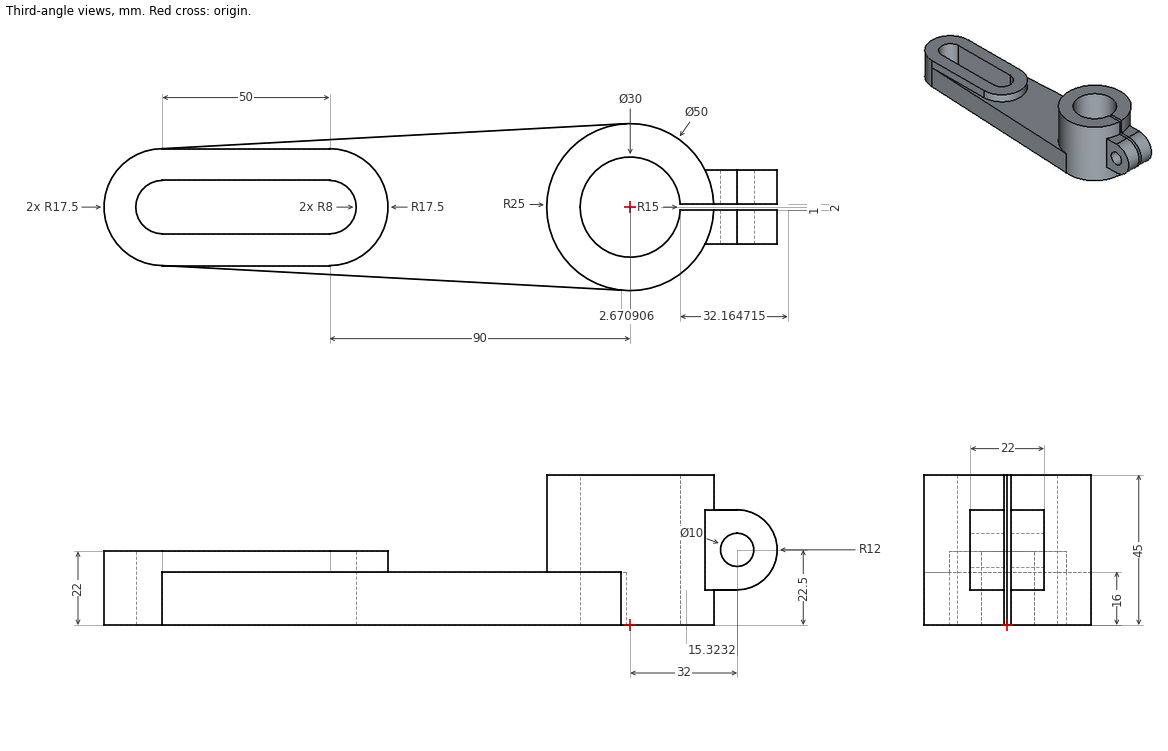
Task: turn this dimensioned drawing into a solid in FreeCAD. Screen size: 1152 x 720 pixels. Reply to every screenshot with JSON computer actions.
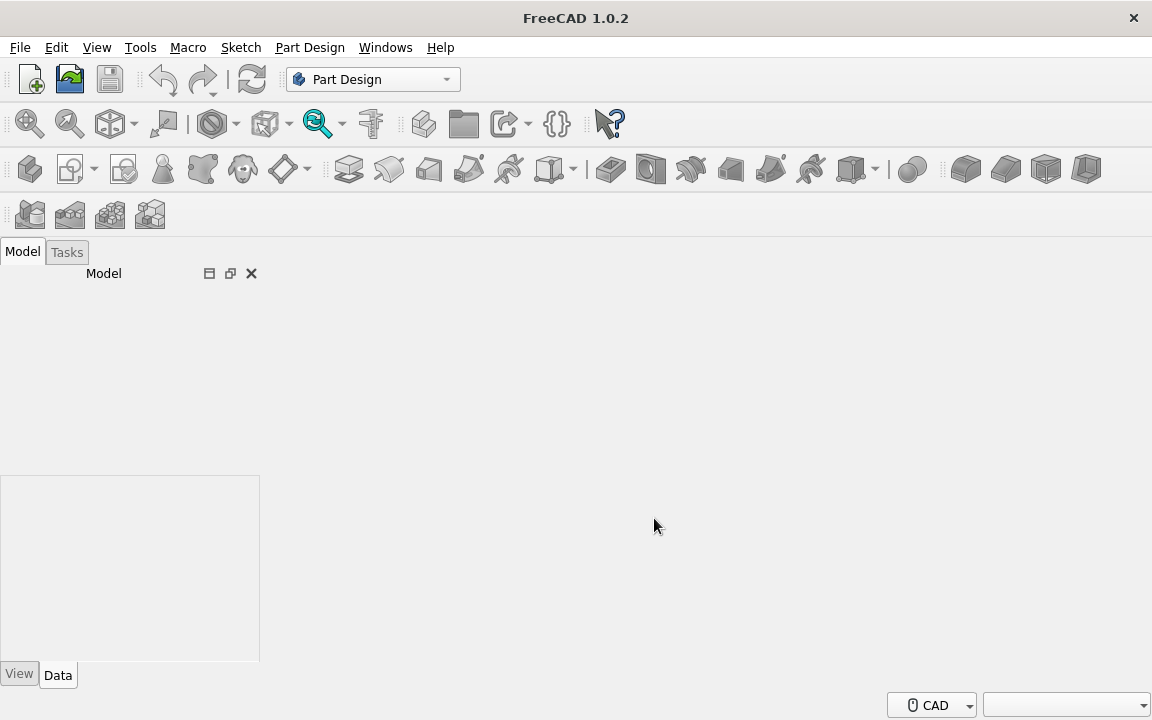
{"action": "left_click", "coordinate": [30, 80]}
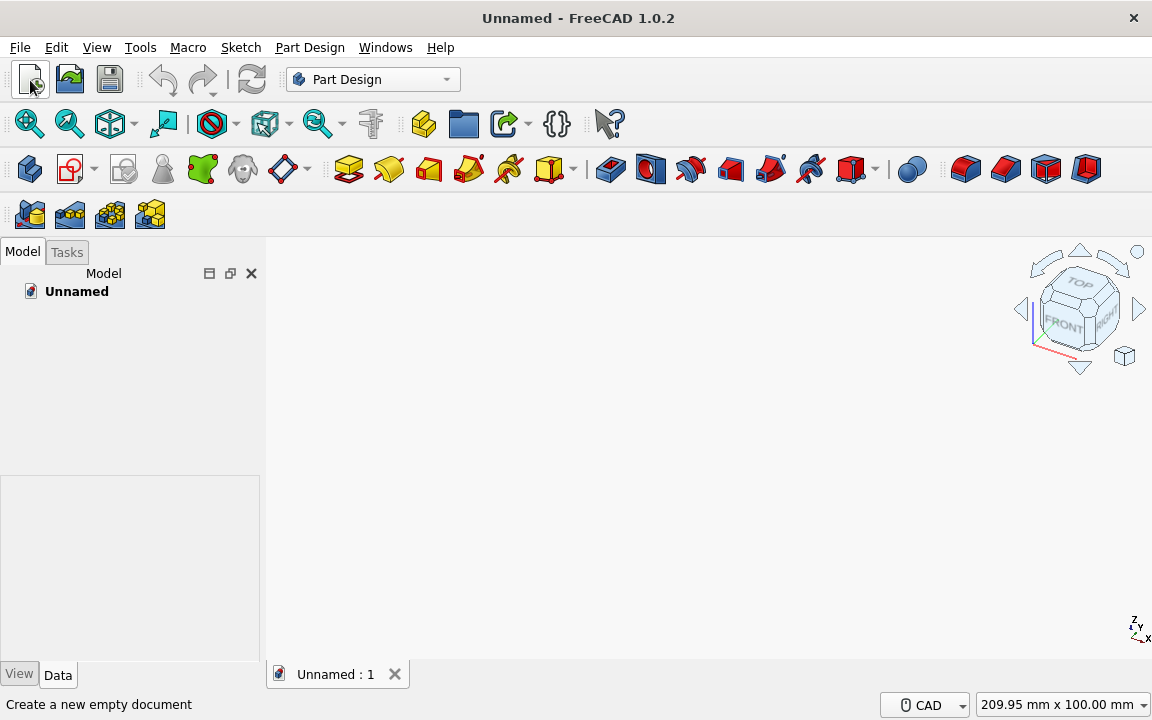
{"action": "left_click", "coordinate": [70, 170]}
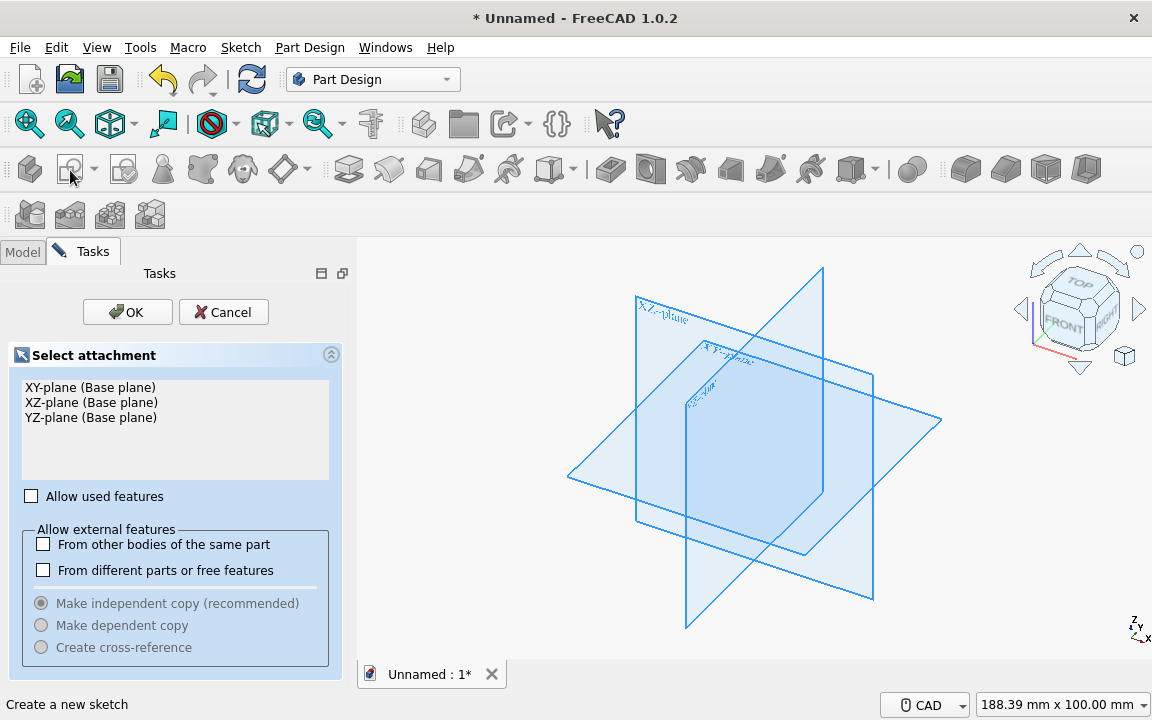
{"action": "left_click", "coordinate": [82, 388]}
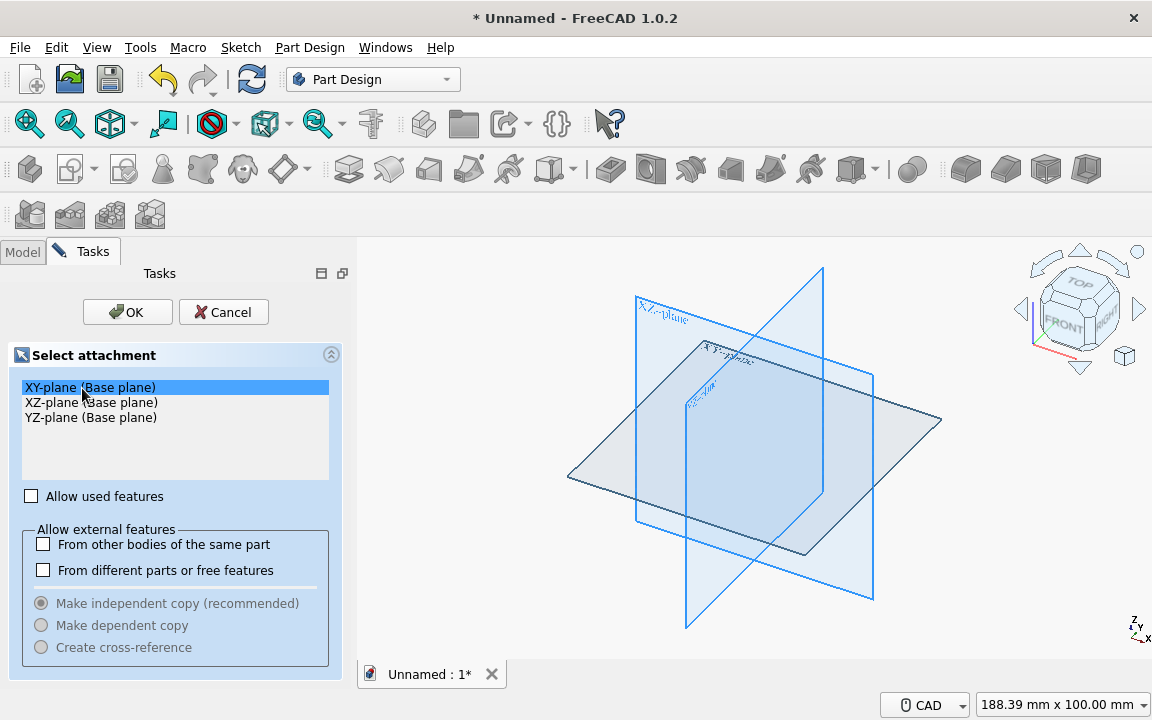
{"action": "left_click", "coordinate": [128, 312]}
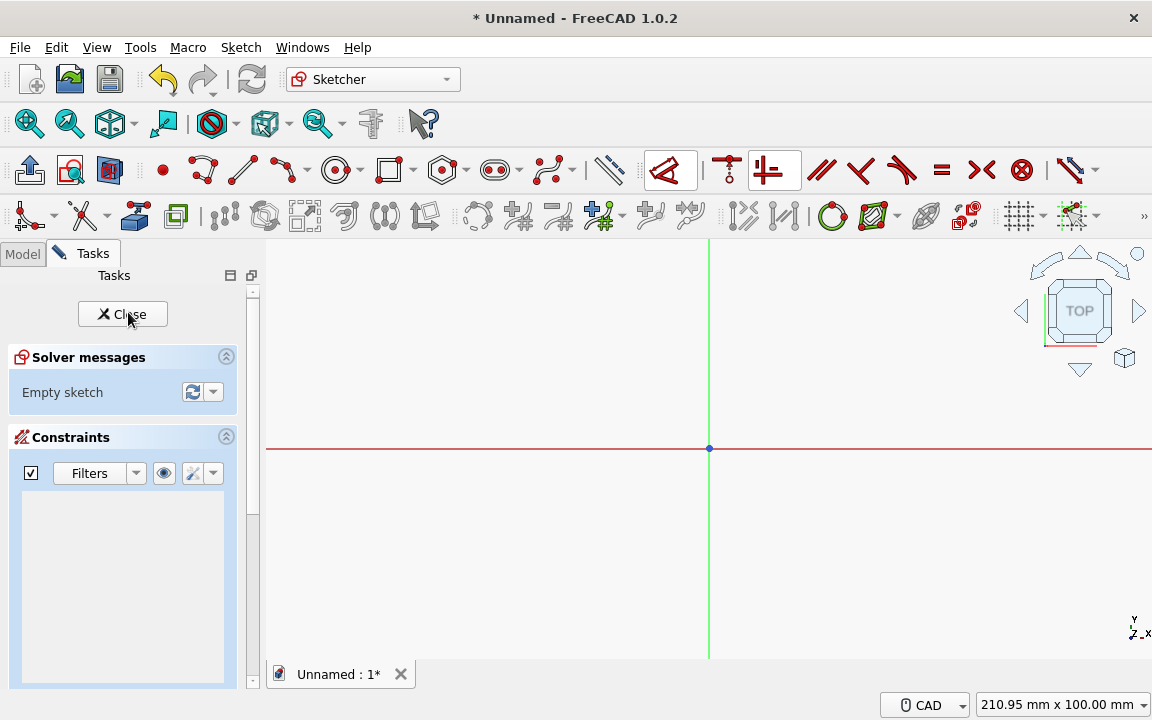
{"action": "left_click", "coordinate": [336, 170]}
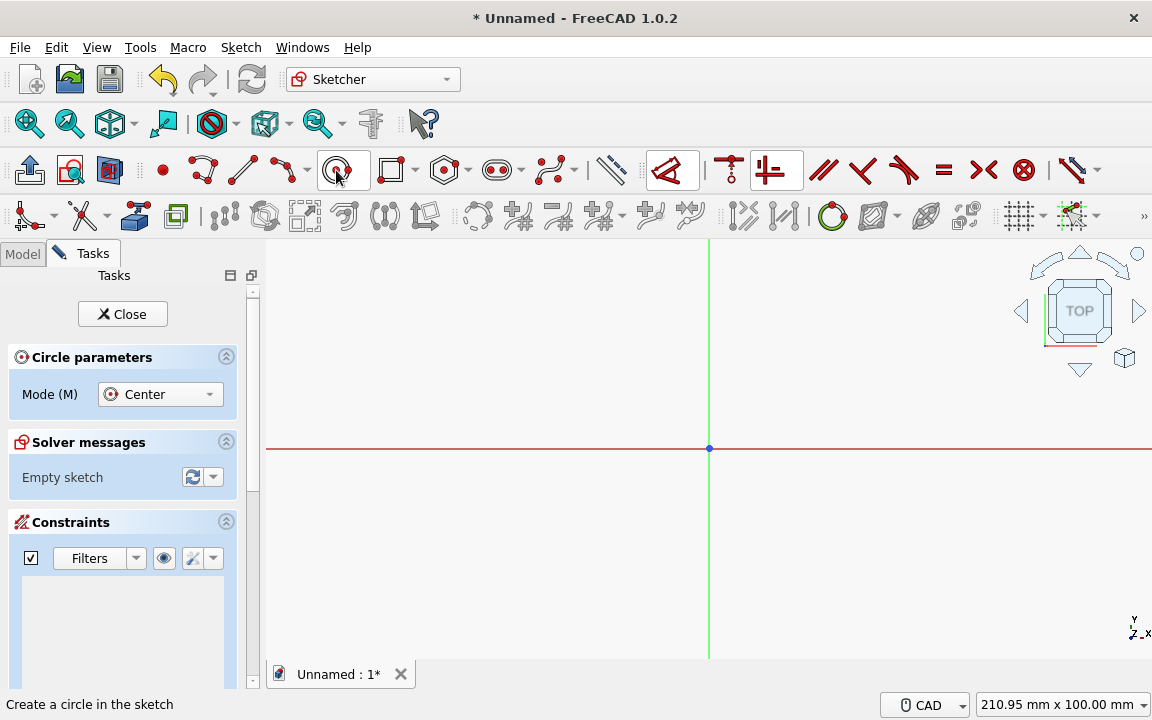
{"action": "left_click", "coordinate": [709, 449]}
{"action": "left_click", "coordinate": [783, 375]}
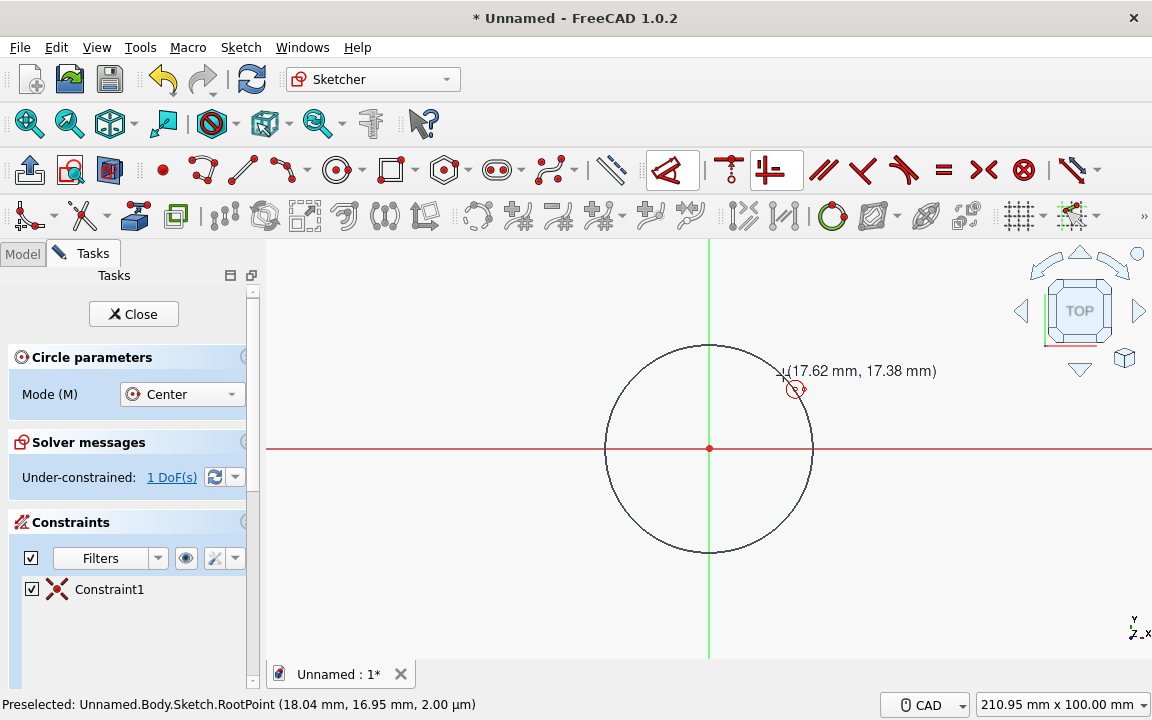
{"action": "left_click", "coordinate": [709, 449]}
{"action": "left_click", "coordinate": [754, 404]}
{"action": "key", "text": "Escape"}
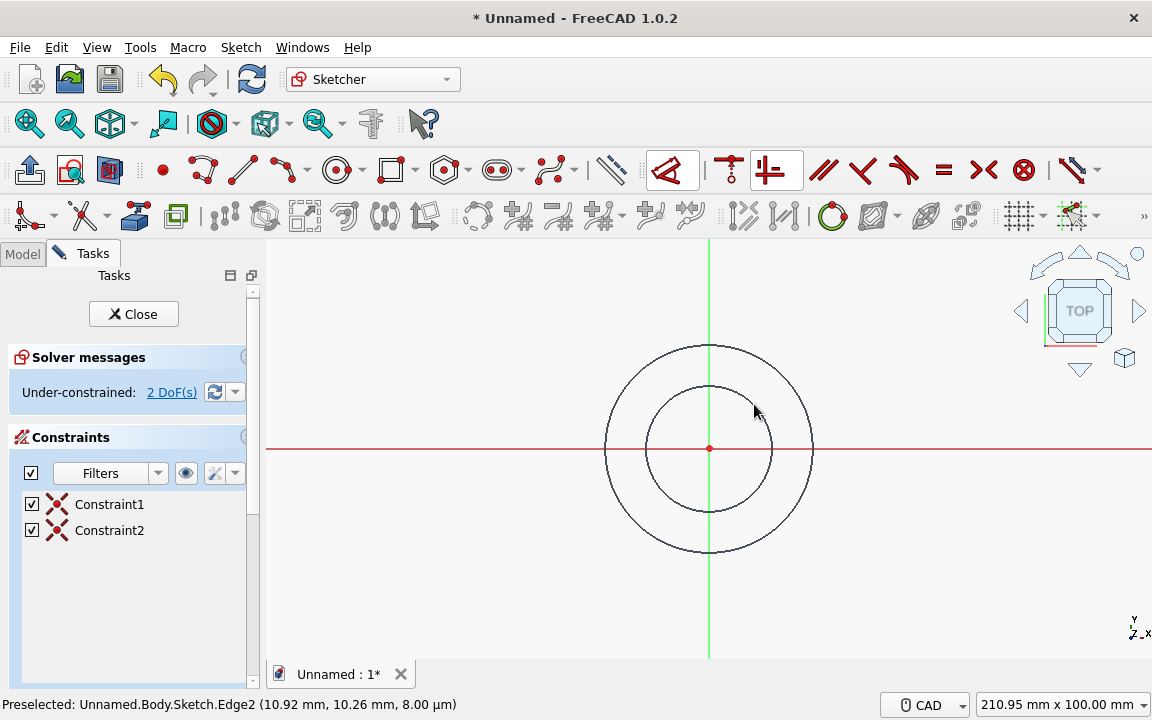
{"action": "left_click", "coordinate": [666, 170]}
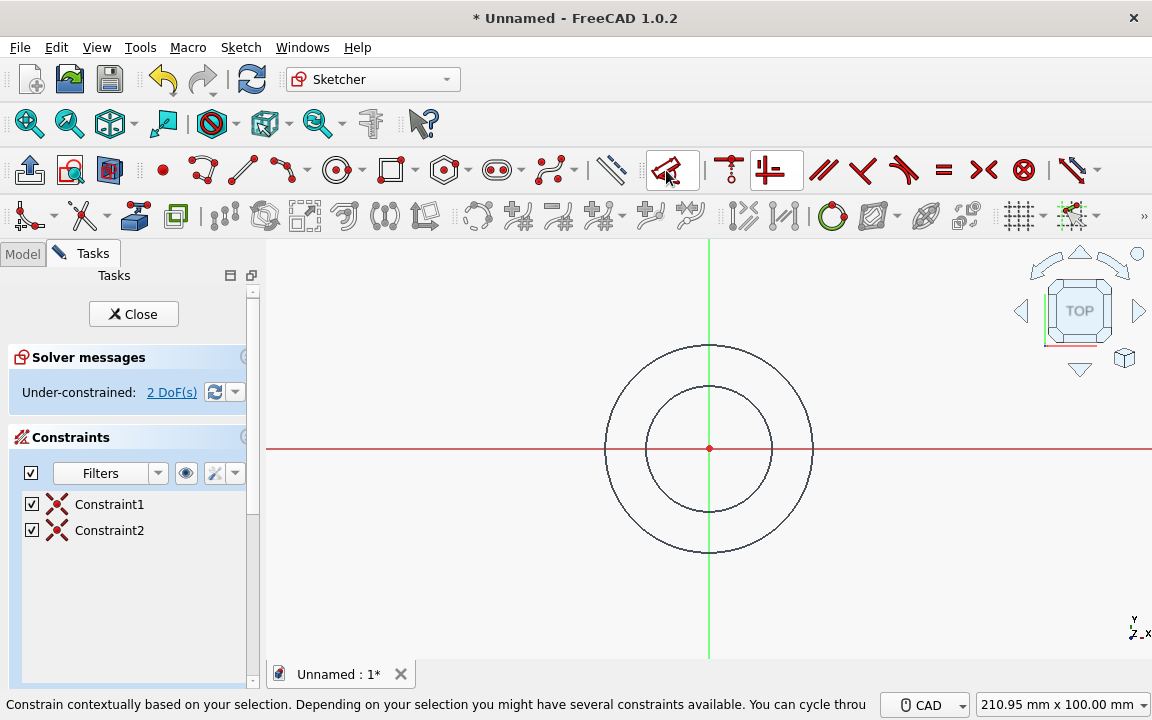
{"action": "left_click", "coordinate": [782, 375]}
{"action": "left_click", "coordinate": [804, 352]}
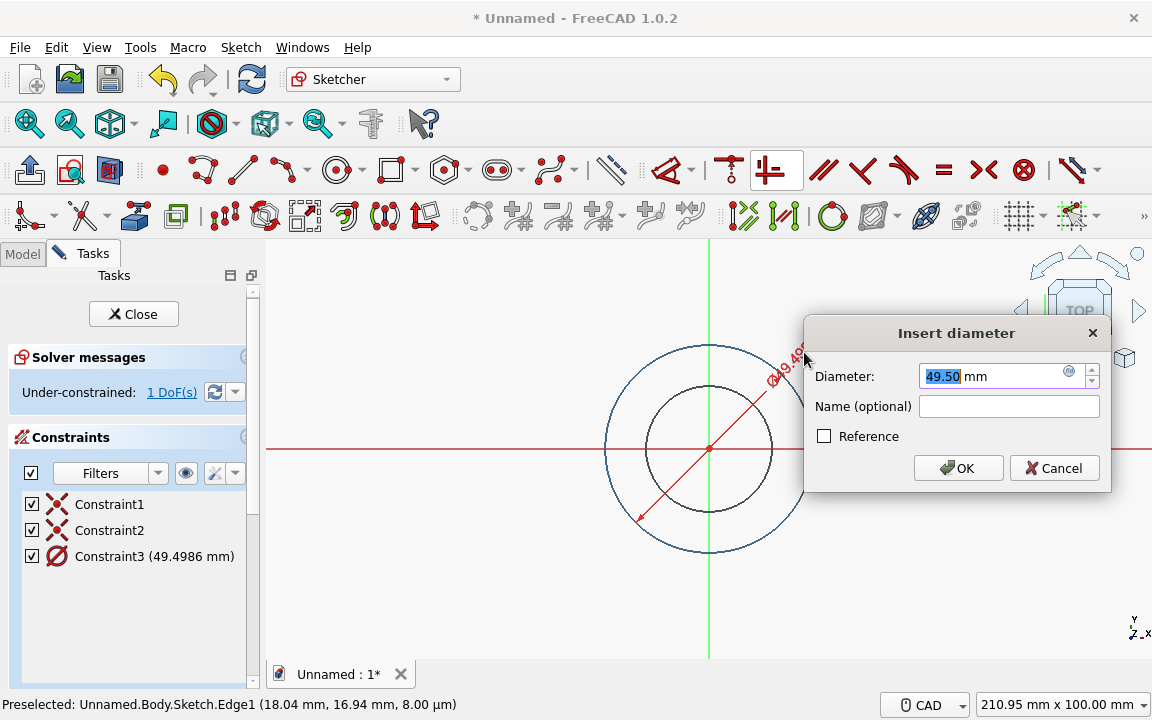
{"action": "type", "text": "50"}
{"action": "key", "text": "Return"}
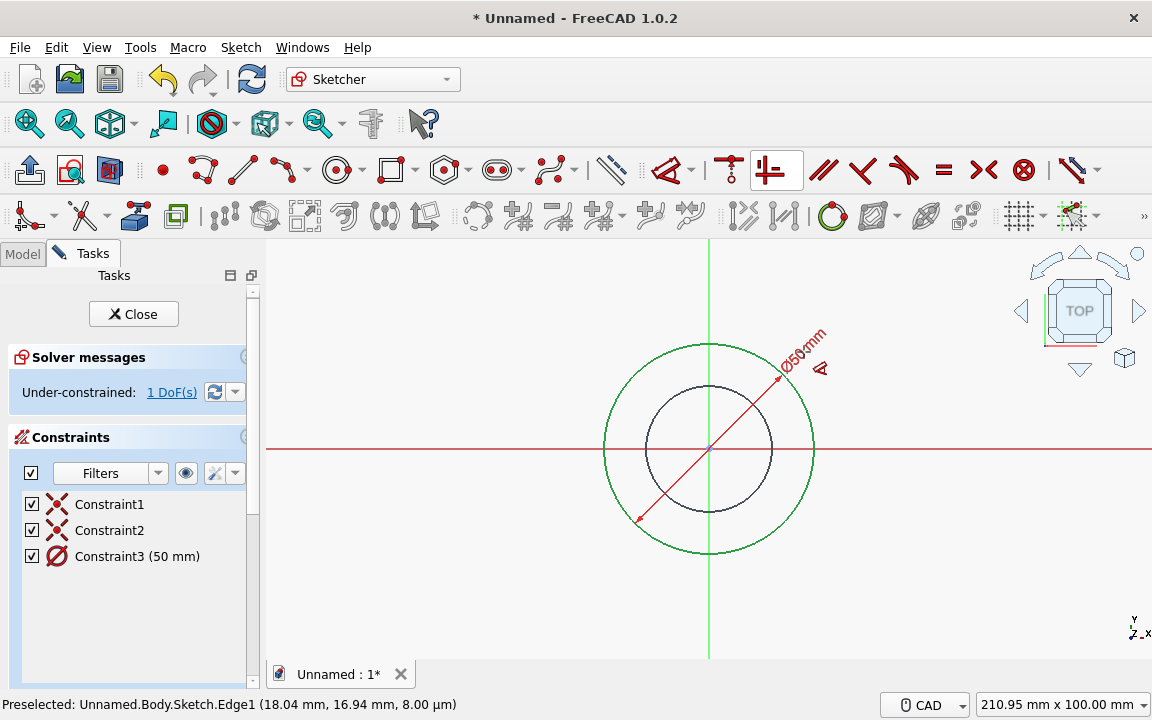
{"action": "left_click", "coordinate": [753, 404]}
{"action": "left_click", "coordinate": [846, 407]}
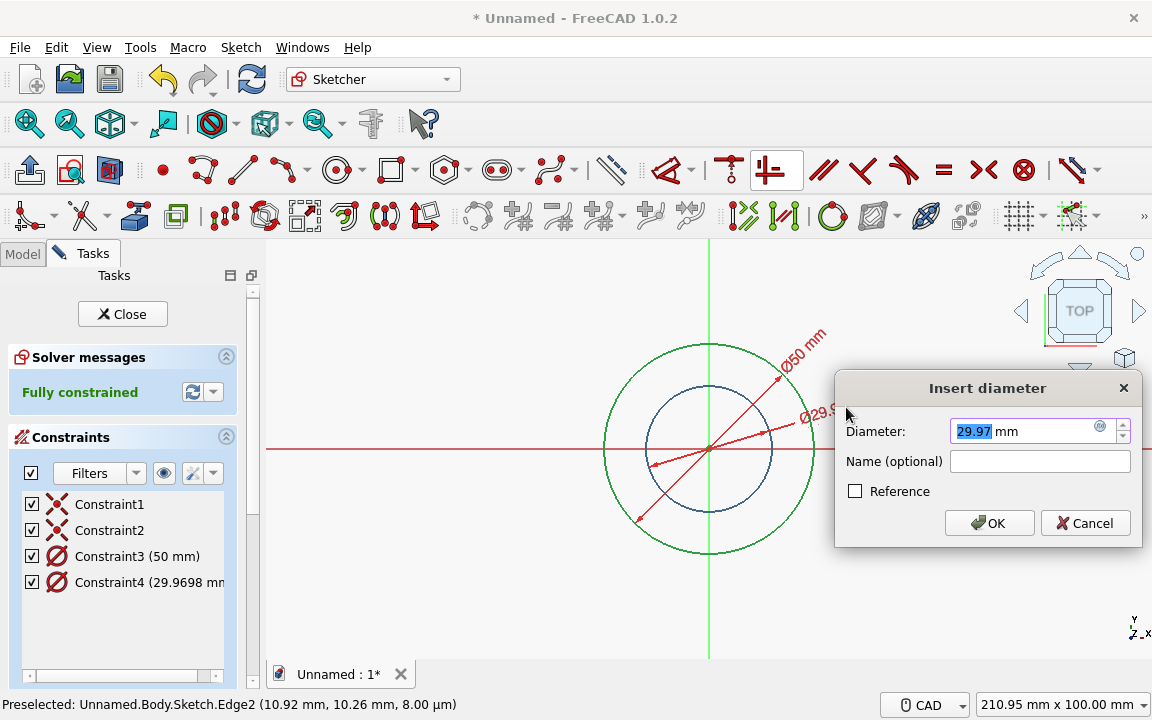
{"action": "type", "text": "30"}
{"action": "key", "text": "Return"}
{"action": "key", "text": "Escape"}